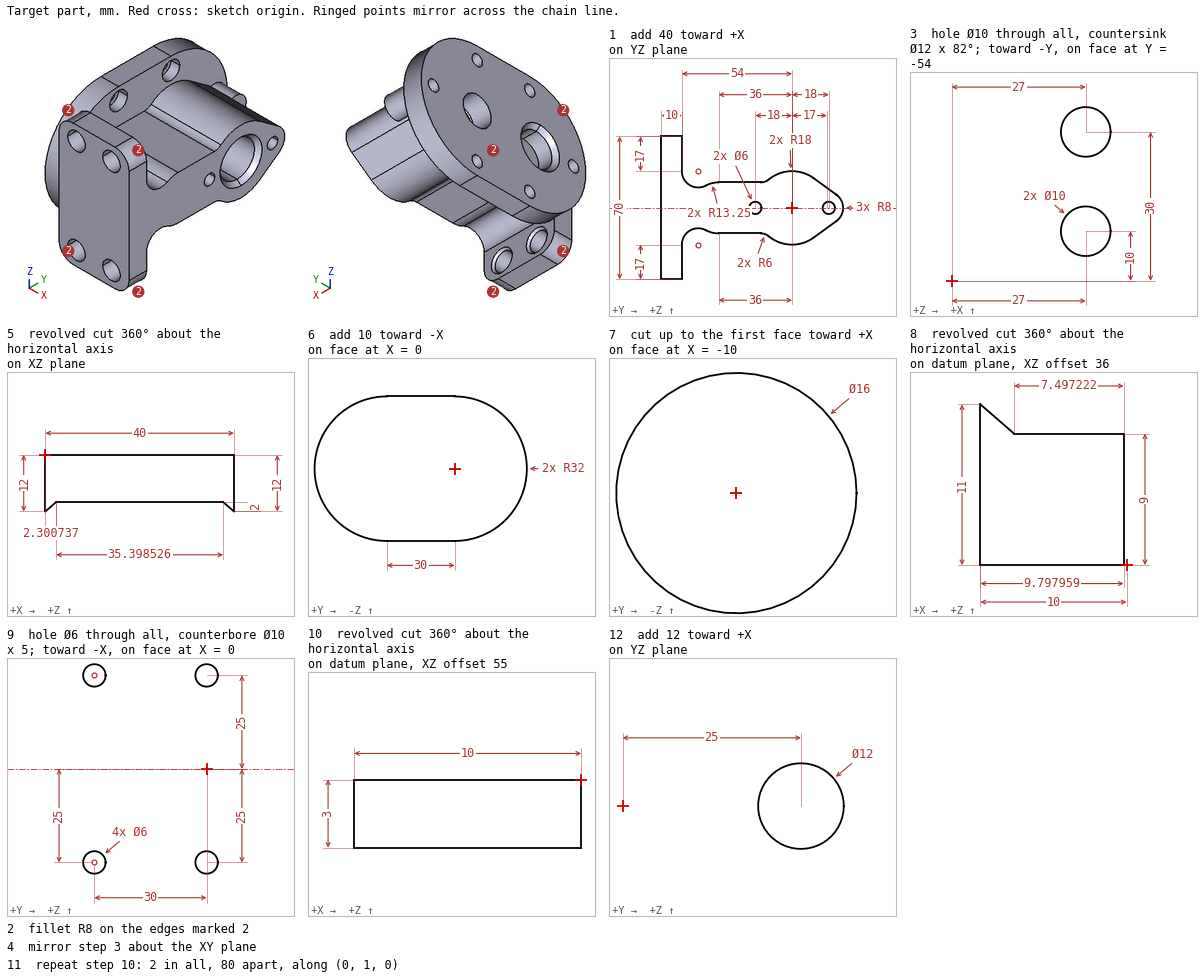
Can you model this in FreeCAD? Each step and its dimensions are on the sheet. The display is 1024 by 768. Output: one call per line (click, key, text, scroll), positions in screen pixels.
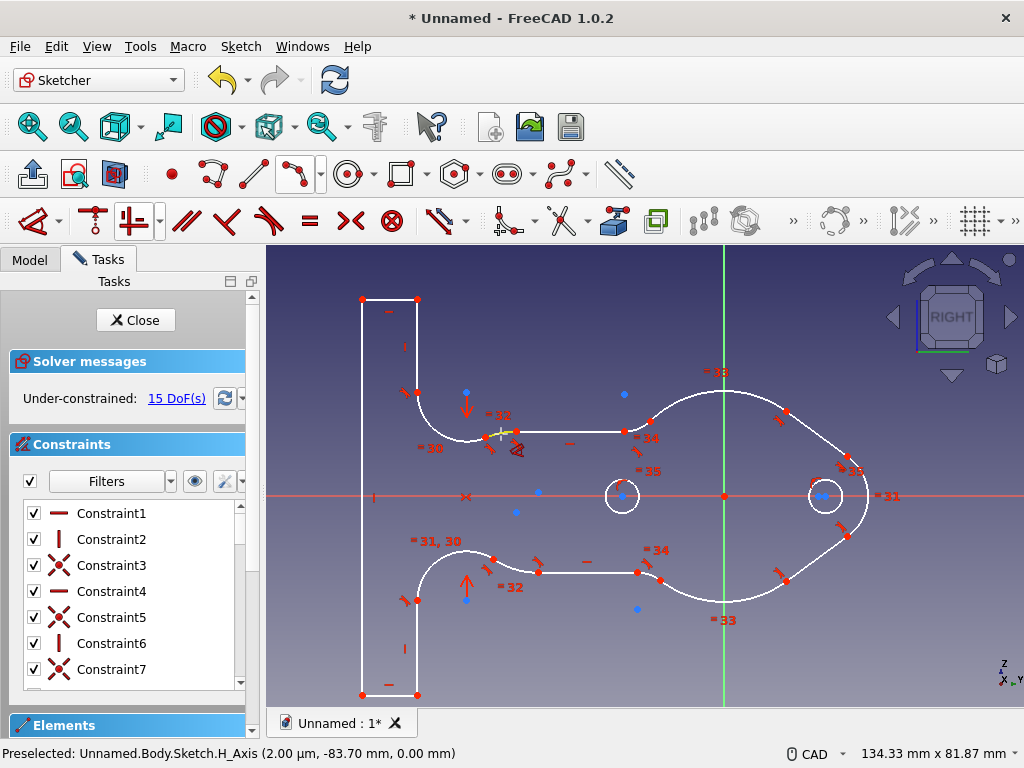
click(501, 433)
click(495, 402)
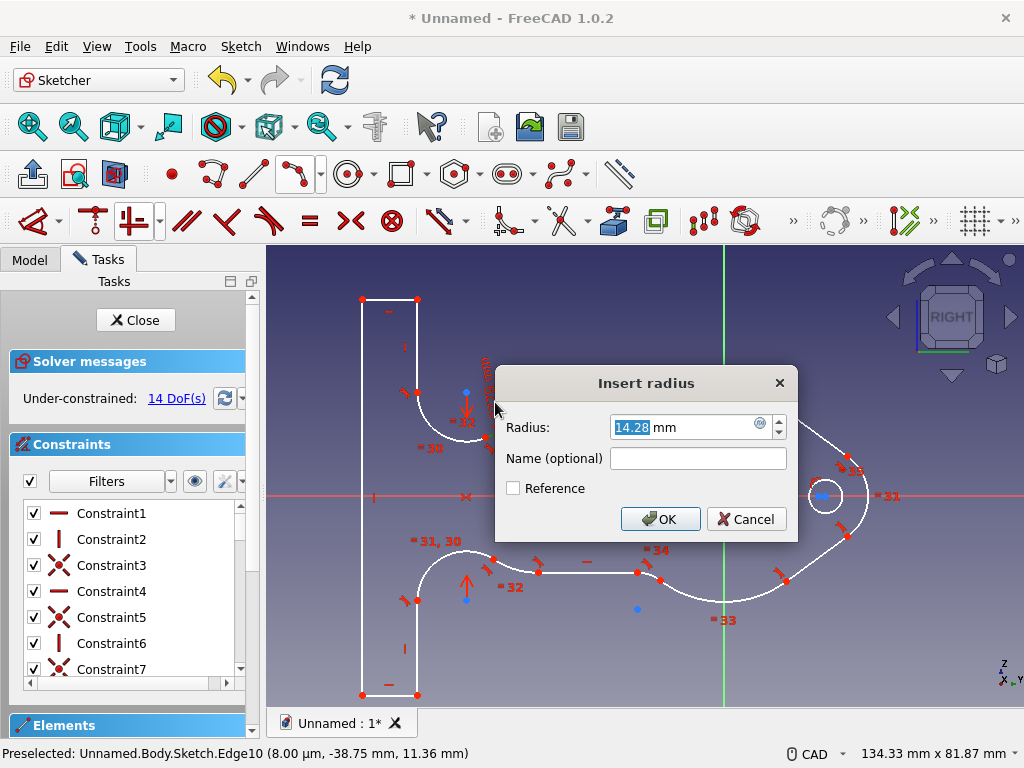
text(13.25)
key(Return)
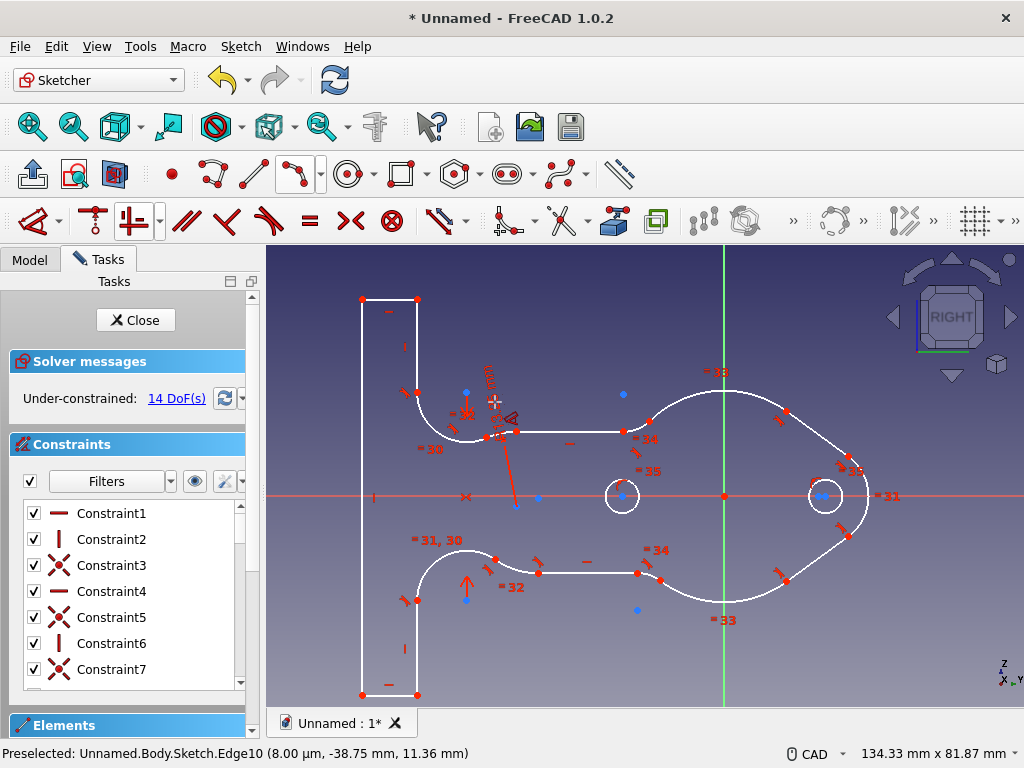
click(426, 420)
click(399, 438)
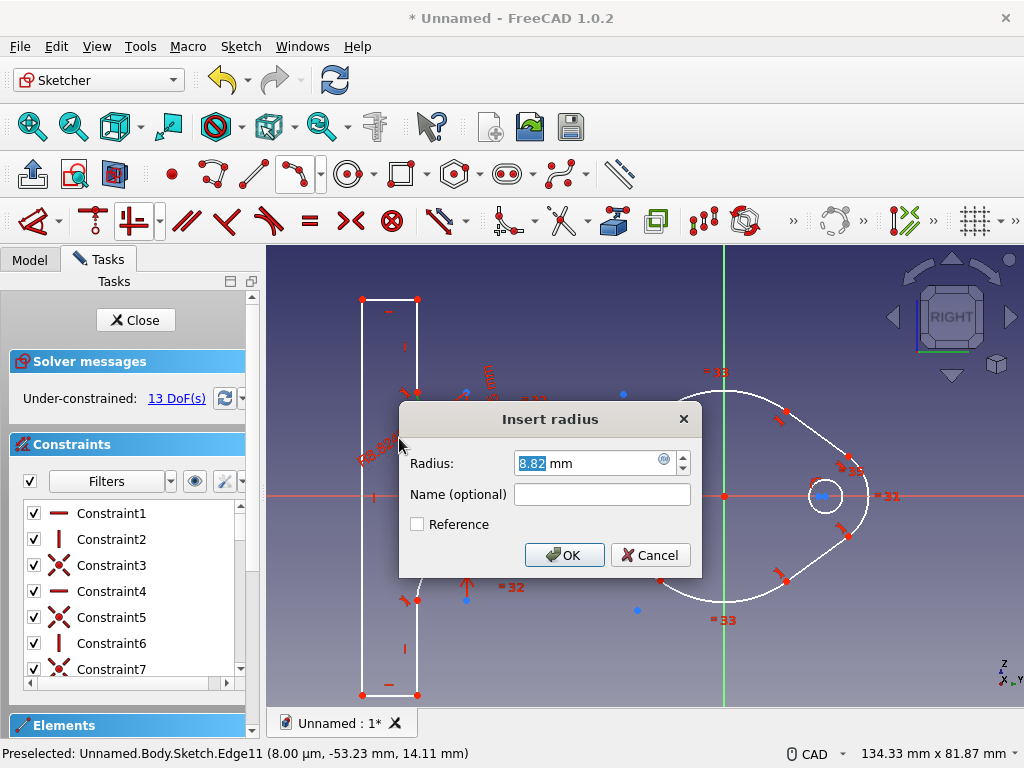
text(8)
key(Return)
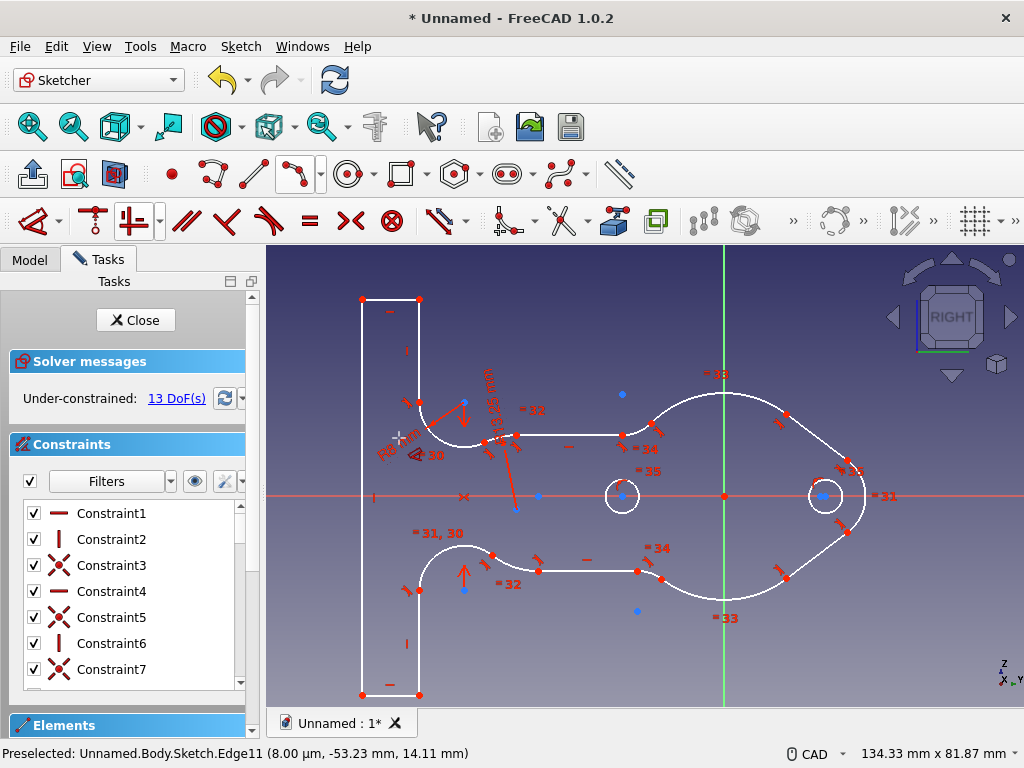
click(650, 573)
click(660, 543)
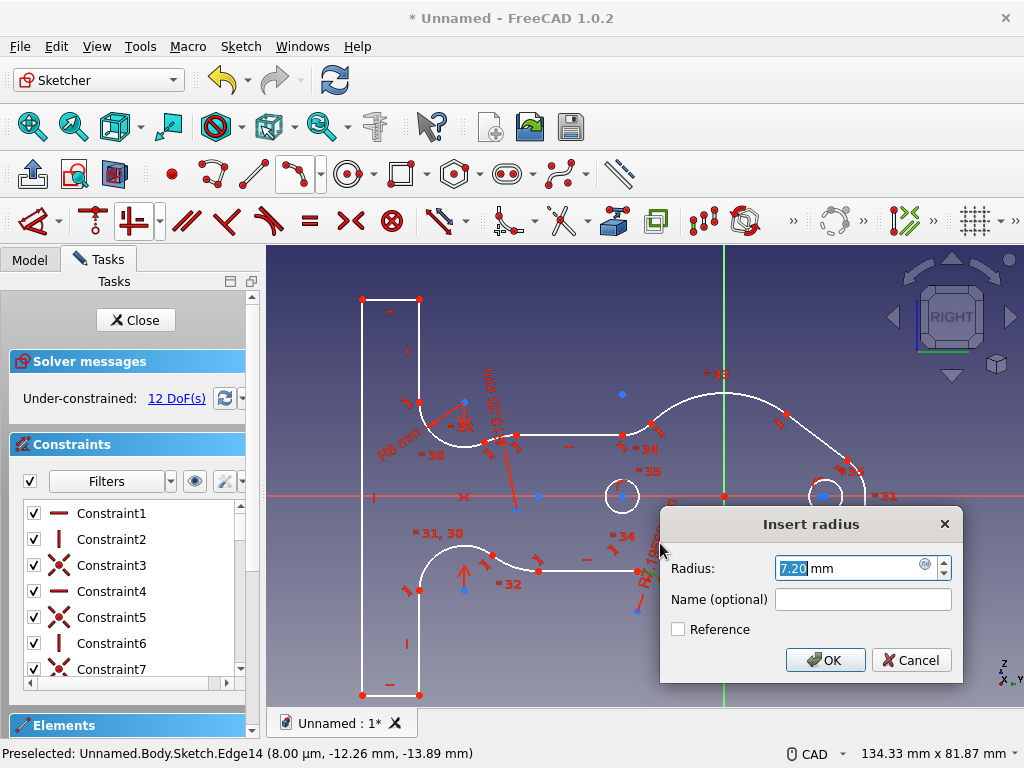
text(6)
key(Return)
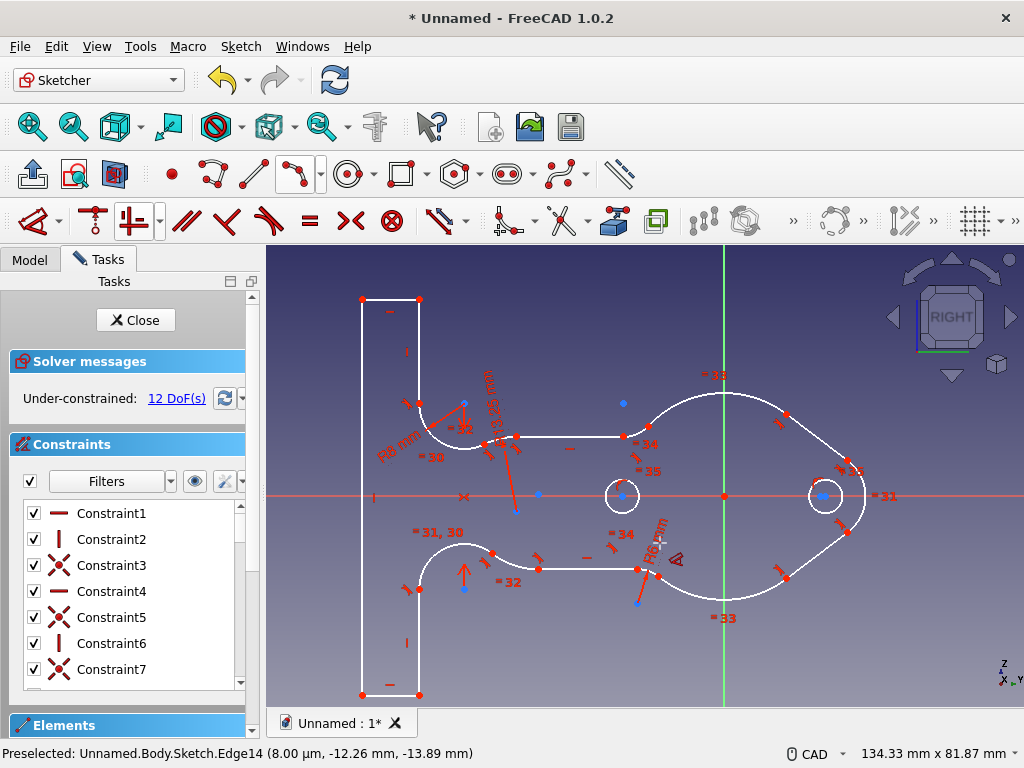
click(695, 596)
click(686, 627)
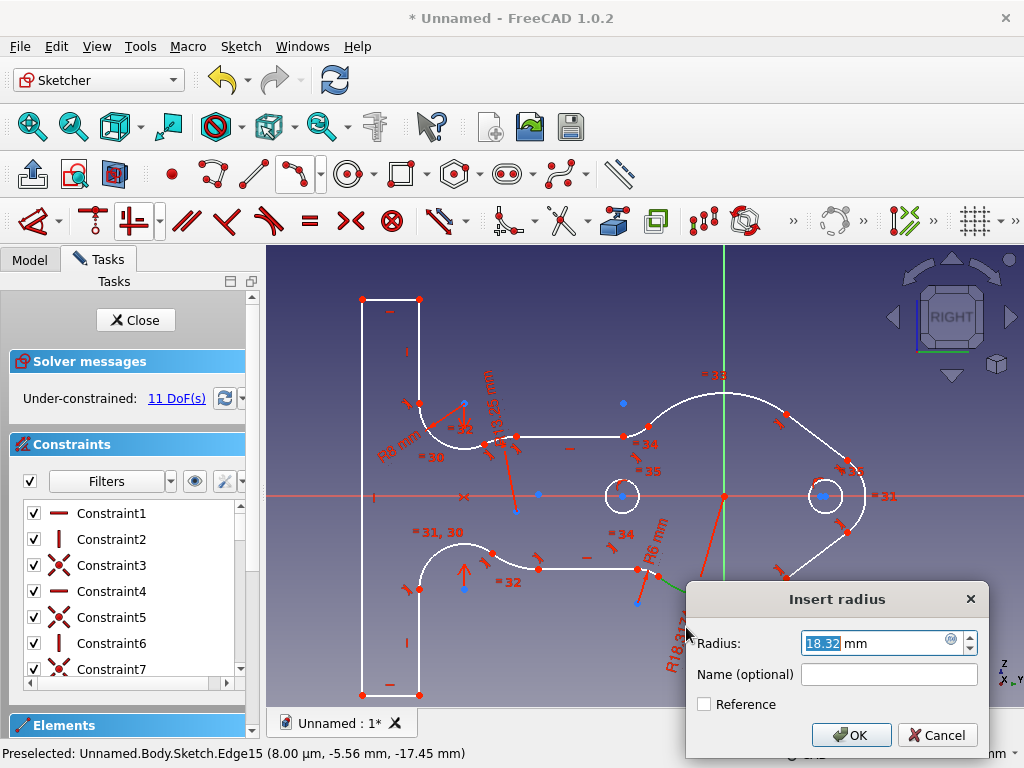
text(18)
key(Return)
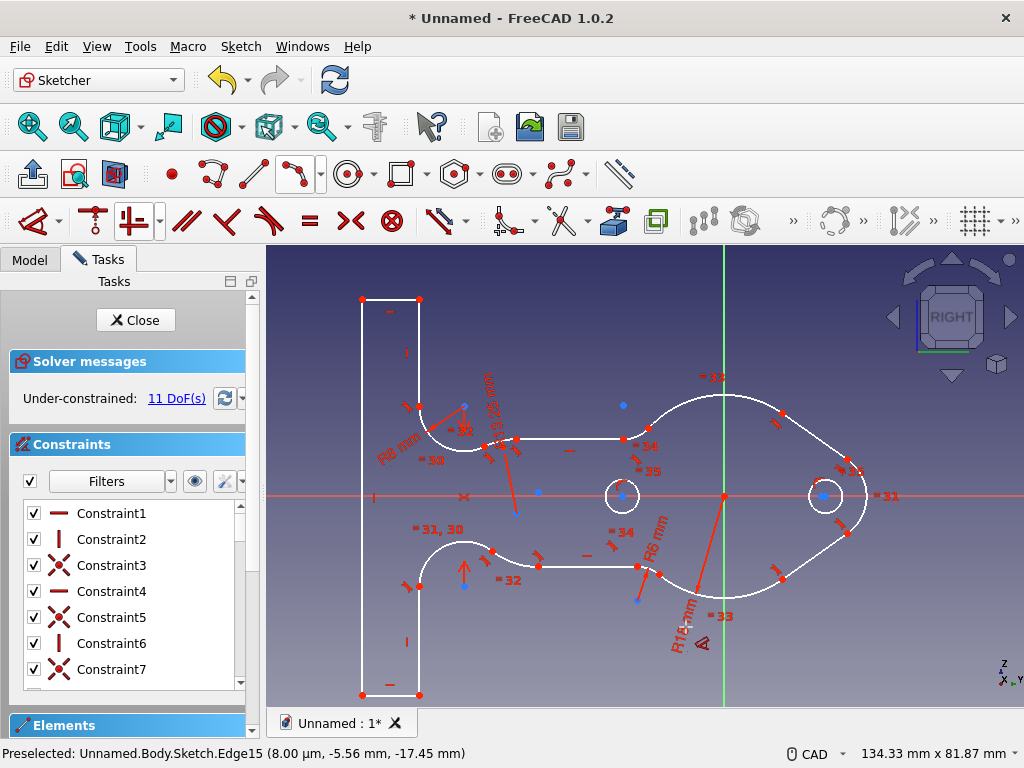
click(634, 485)
click(657, 463)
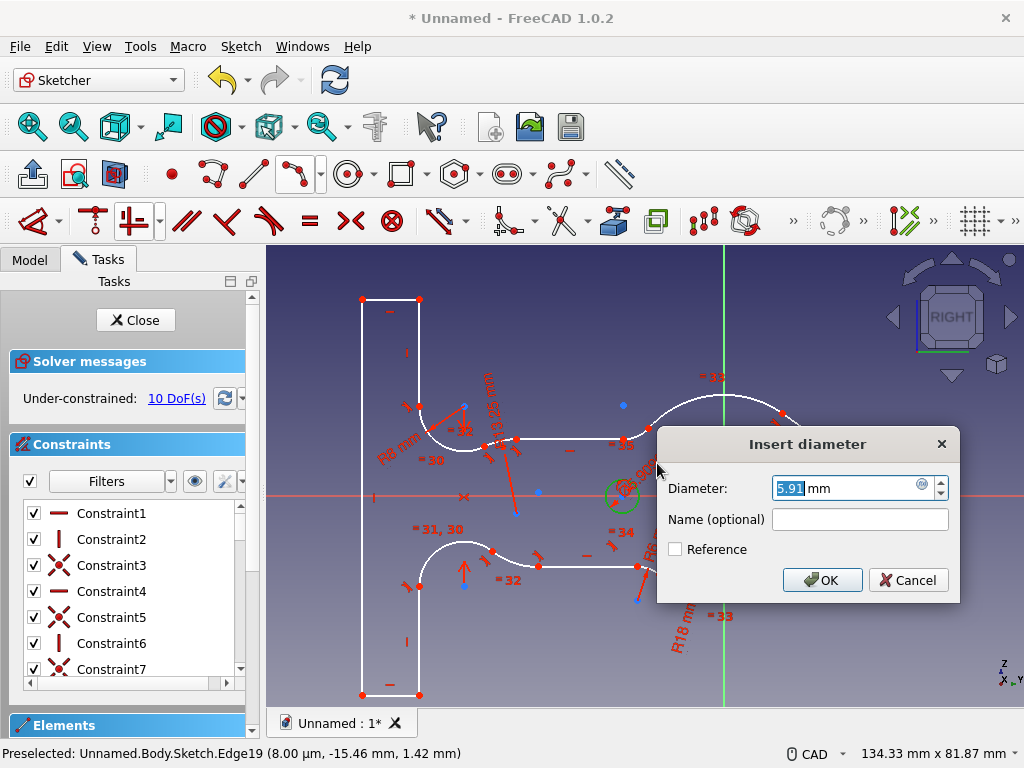
text(6)
key(Return)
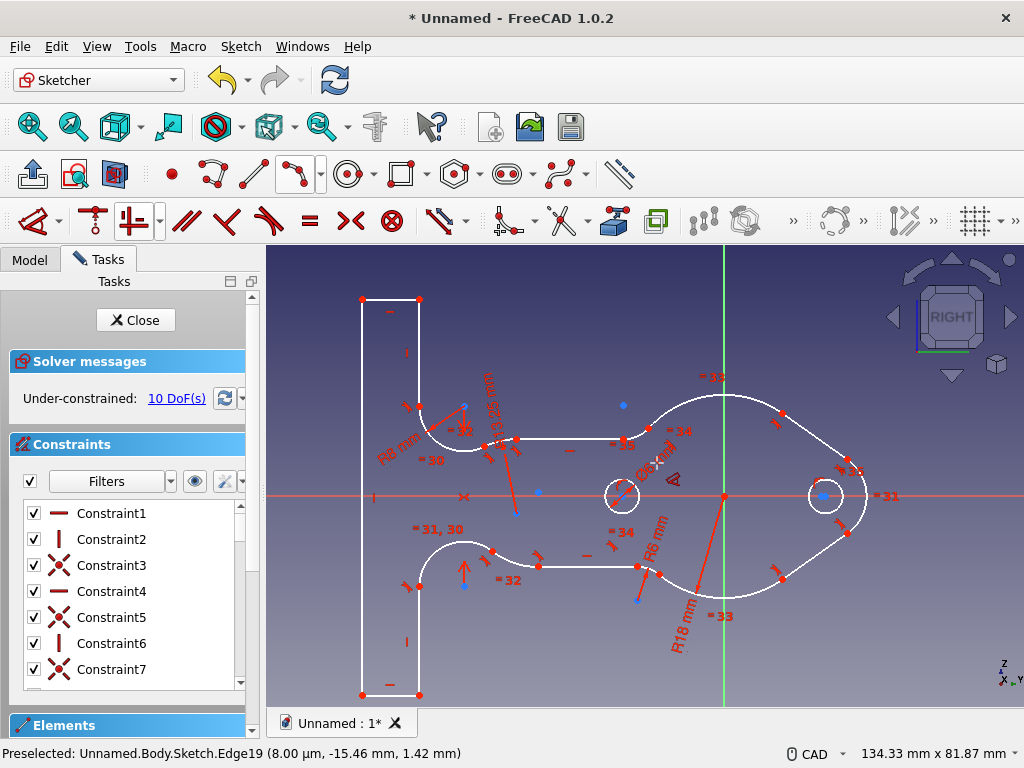
click(419, 374)
click(385, 353)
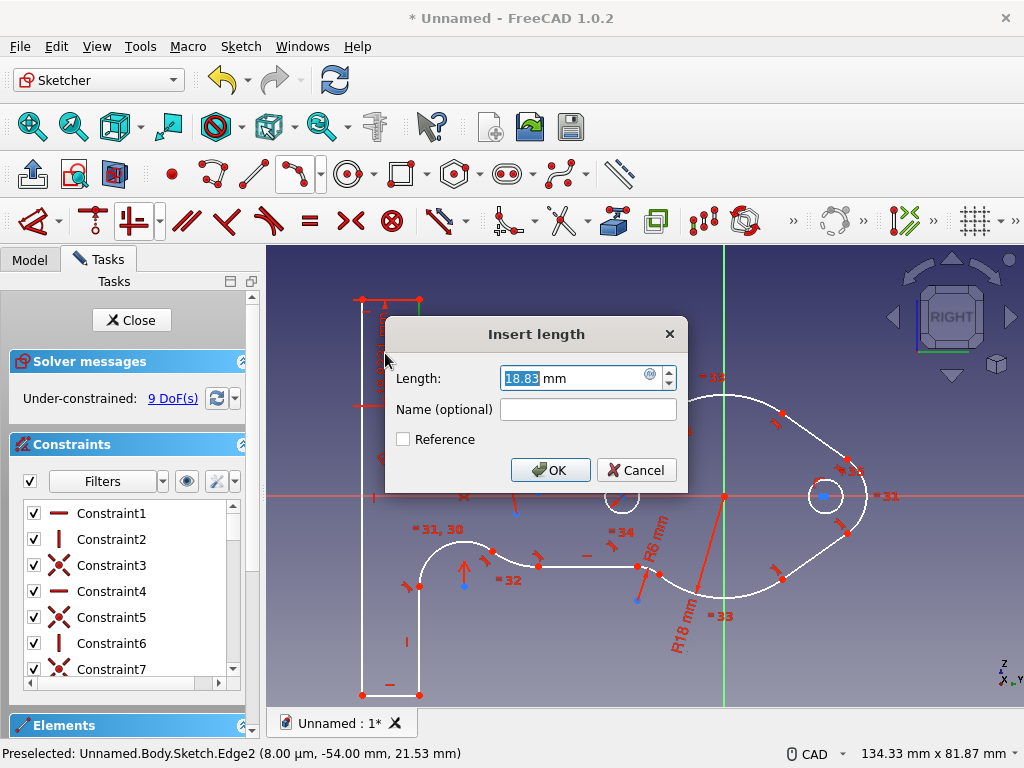
text(17)
key(Return)